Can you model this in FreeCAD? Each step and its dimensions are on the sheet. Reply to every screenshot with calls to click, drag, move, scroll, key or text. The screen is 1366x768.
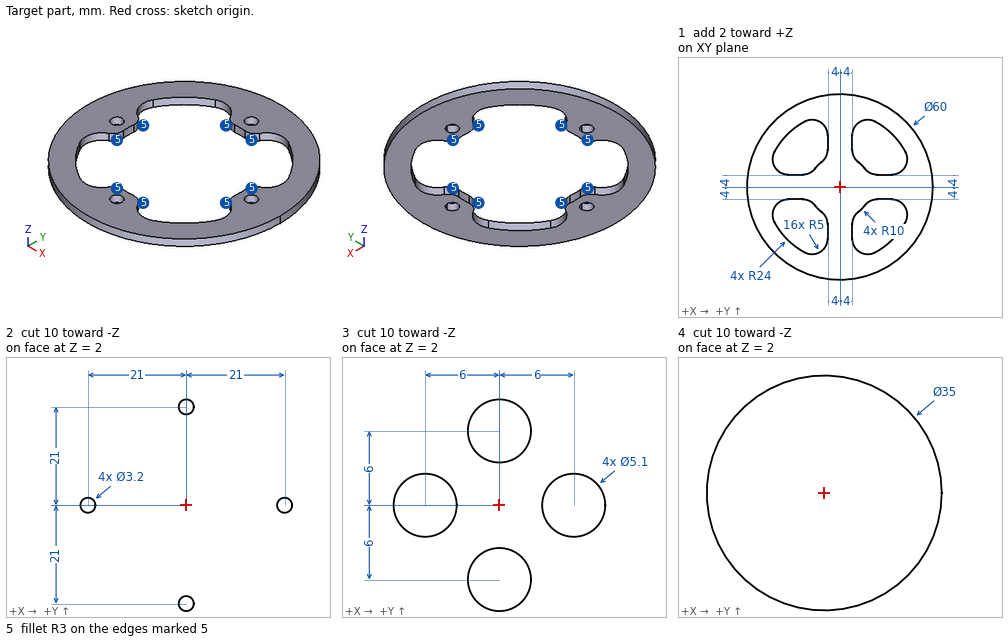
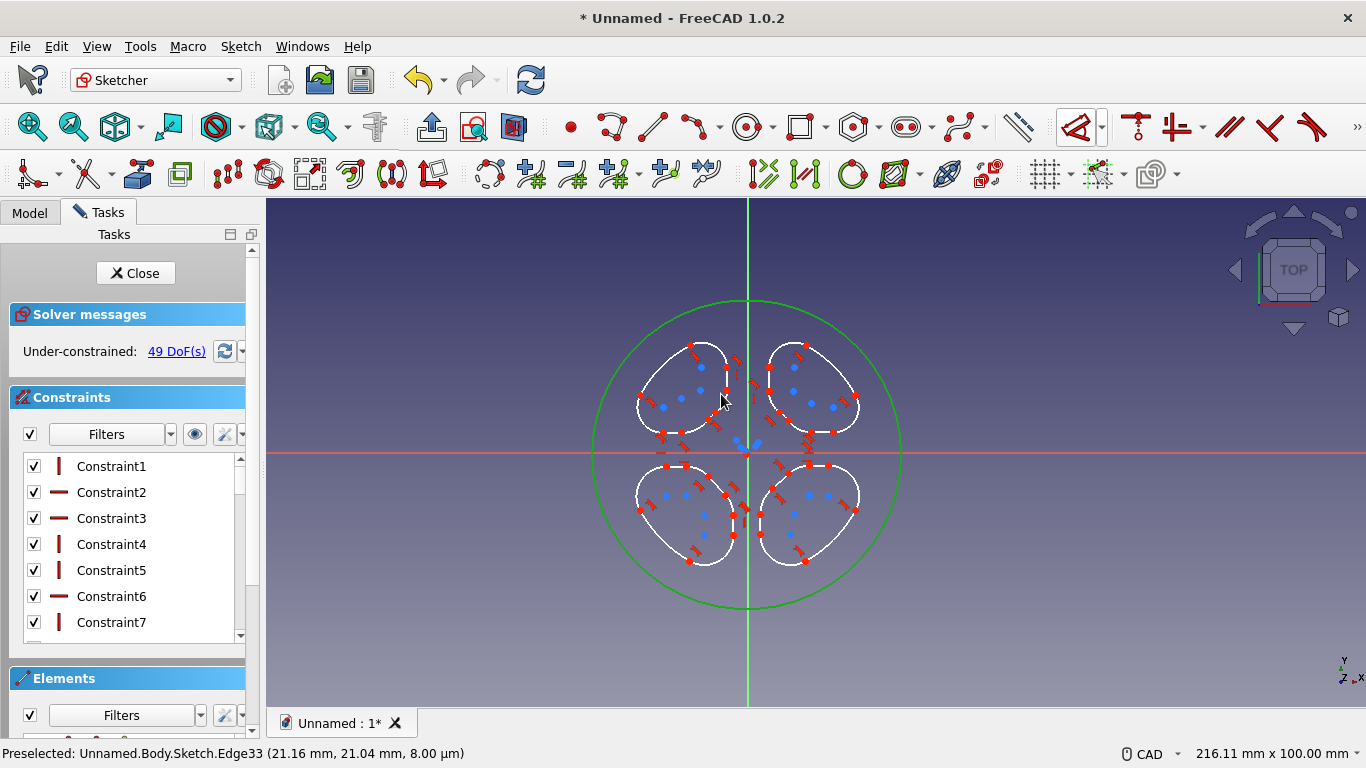
click(652, 529)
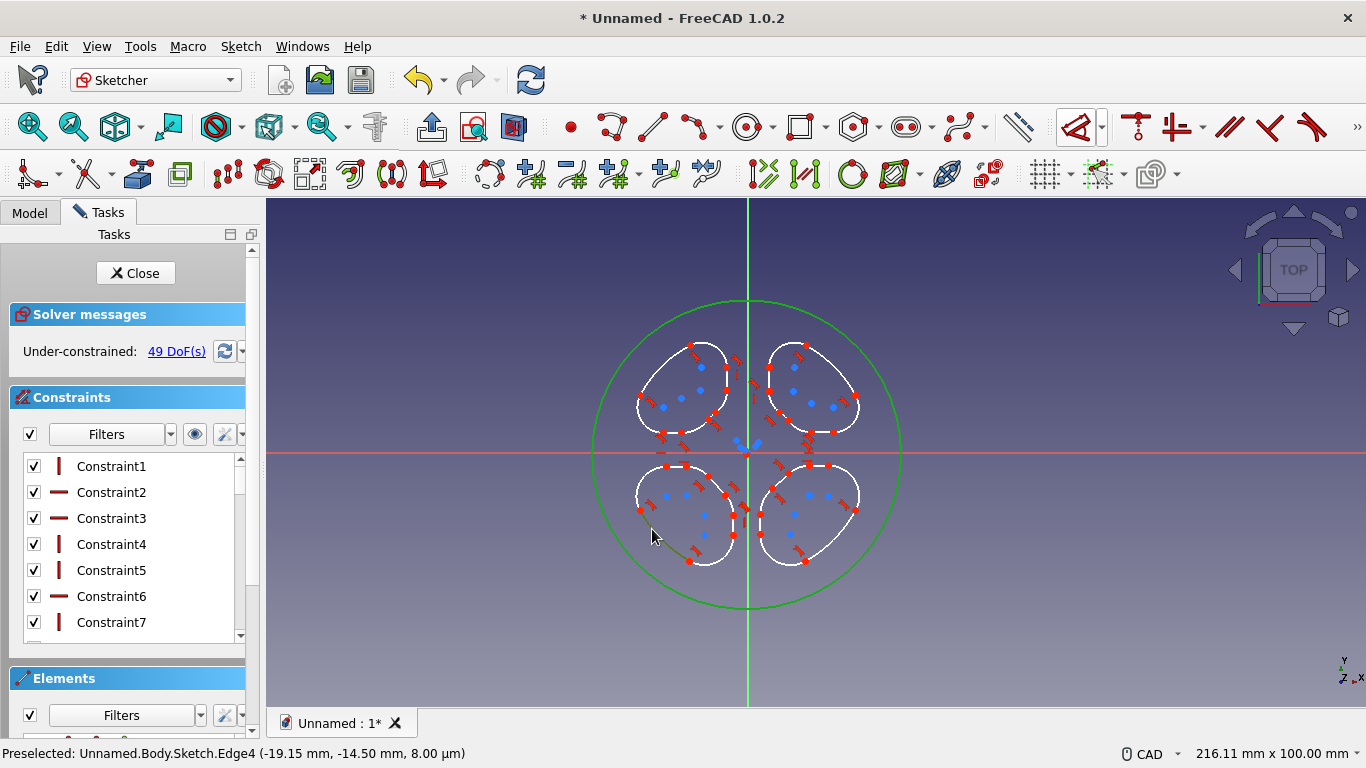
key(c)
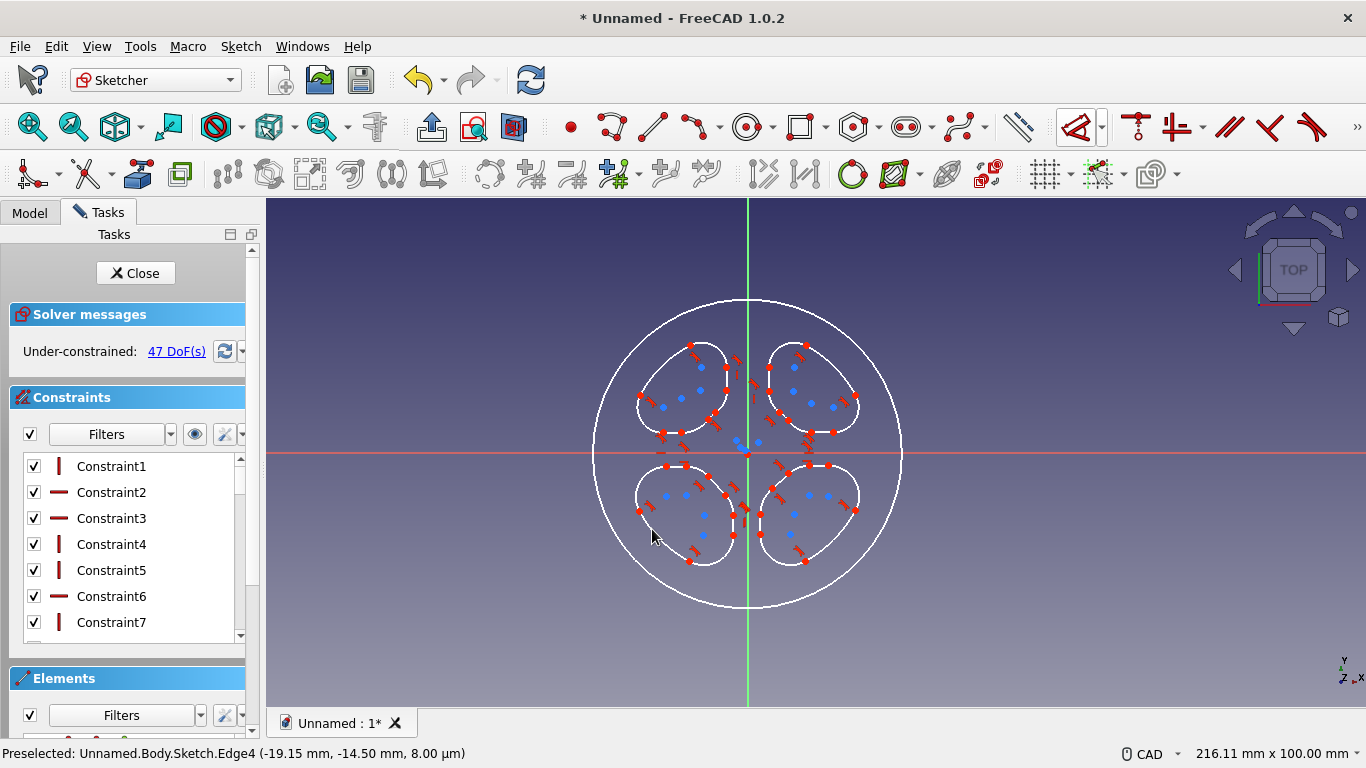
click(856, 344)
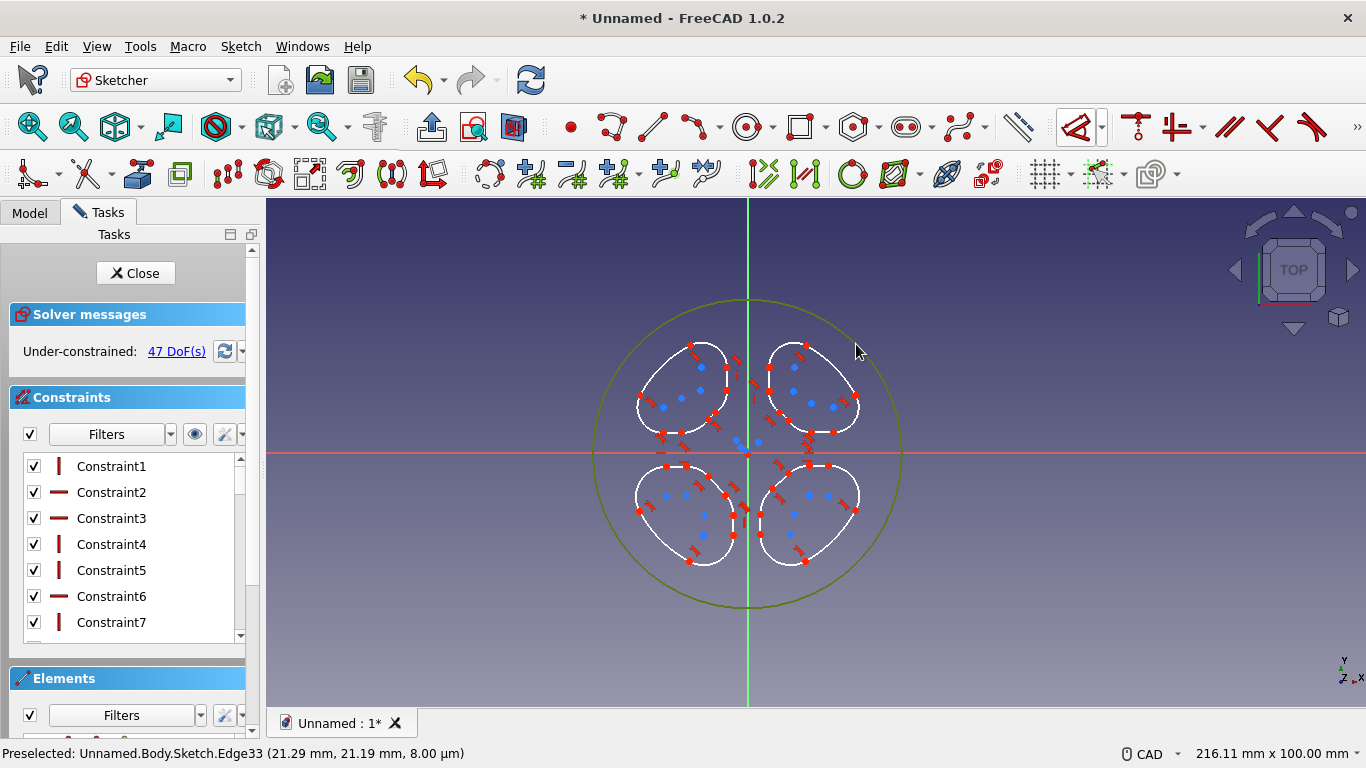
click(717, 486)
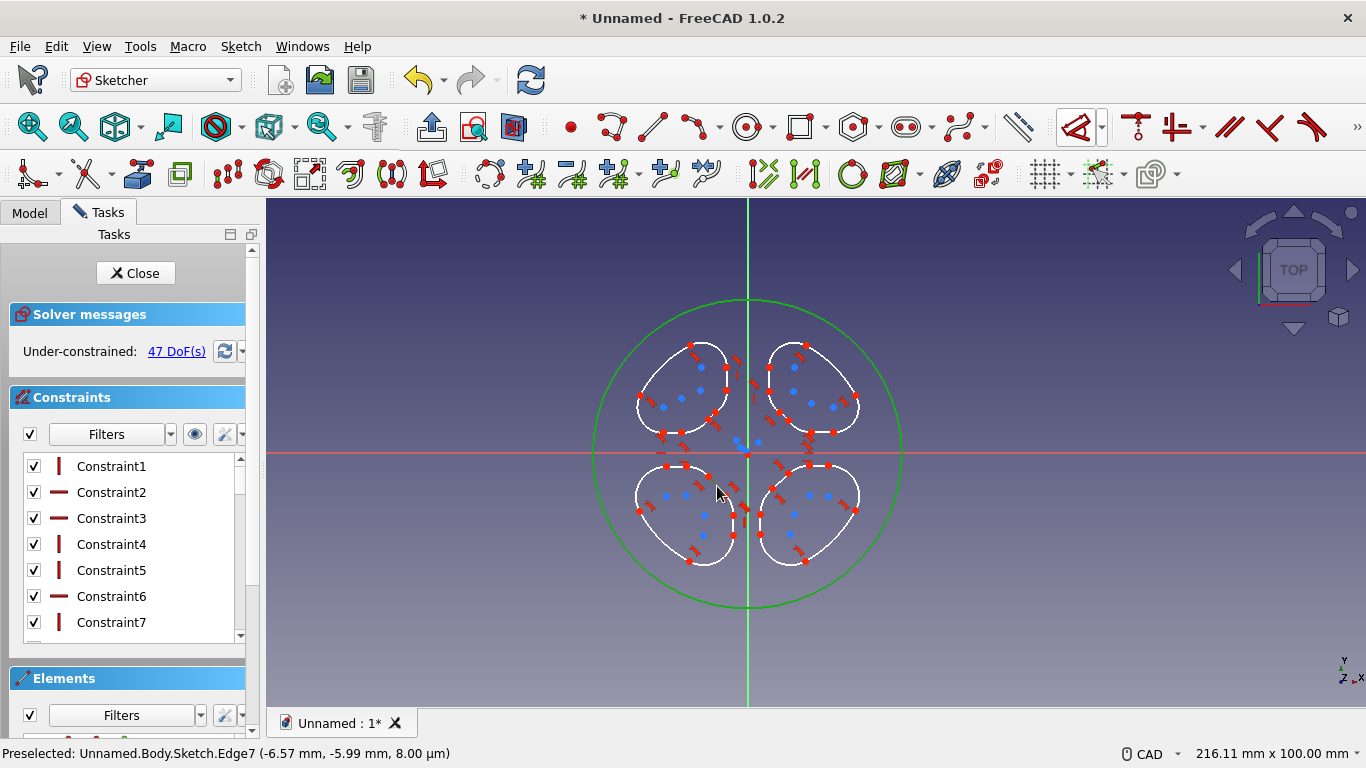
key(c)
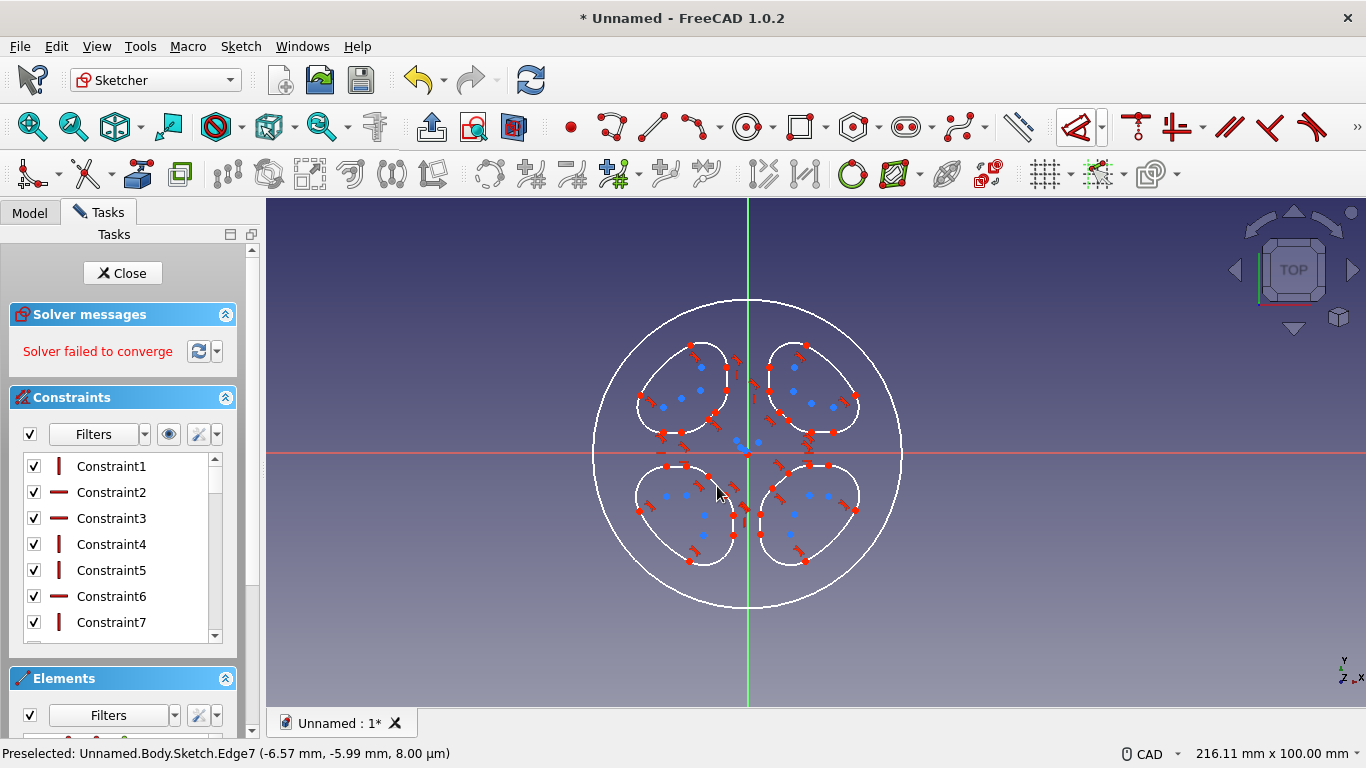
click(856, 344)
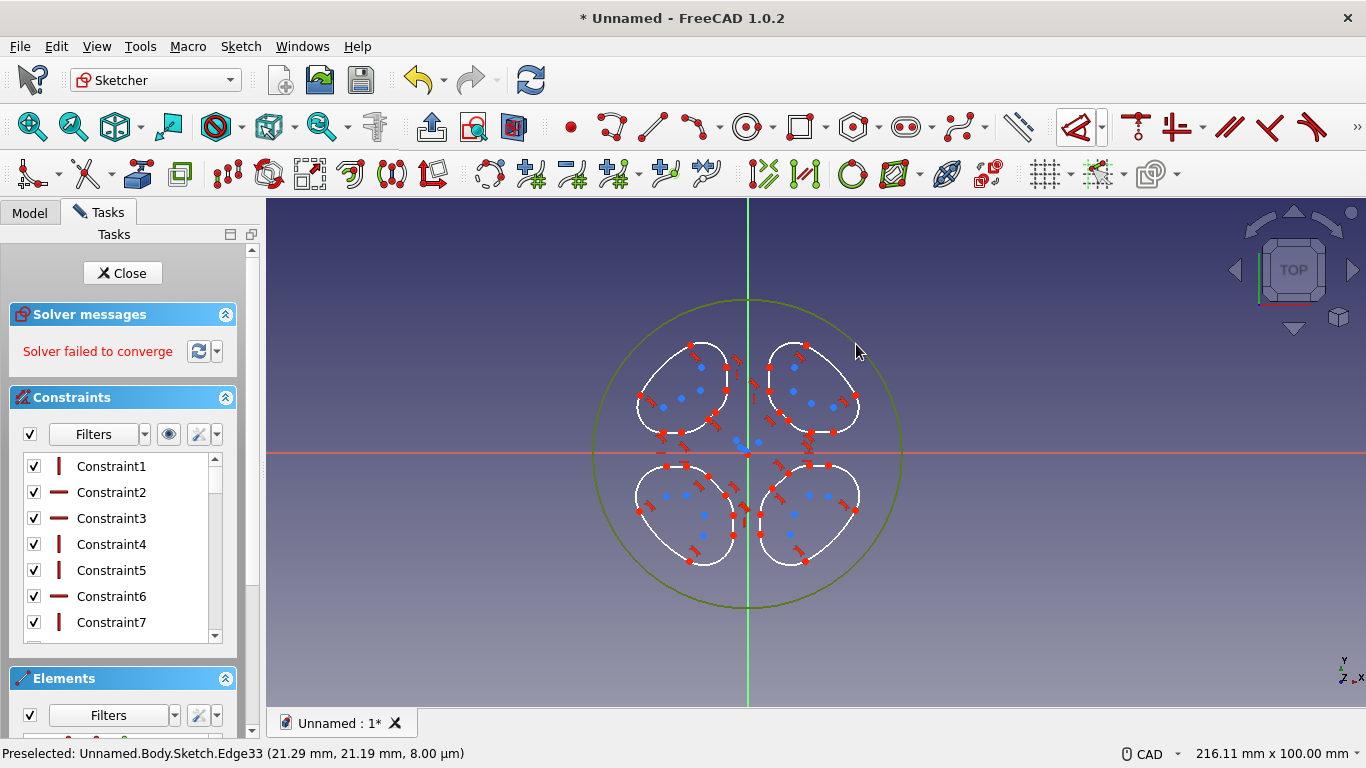
click(823, 549)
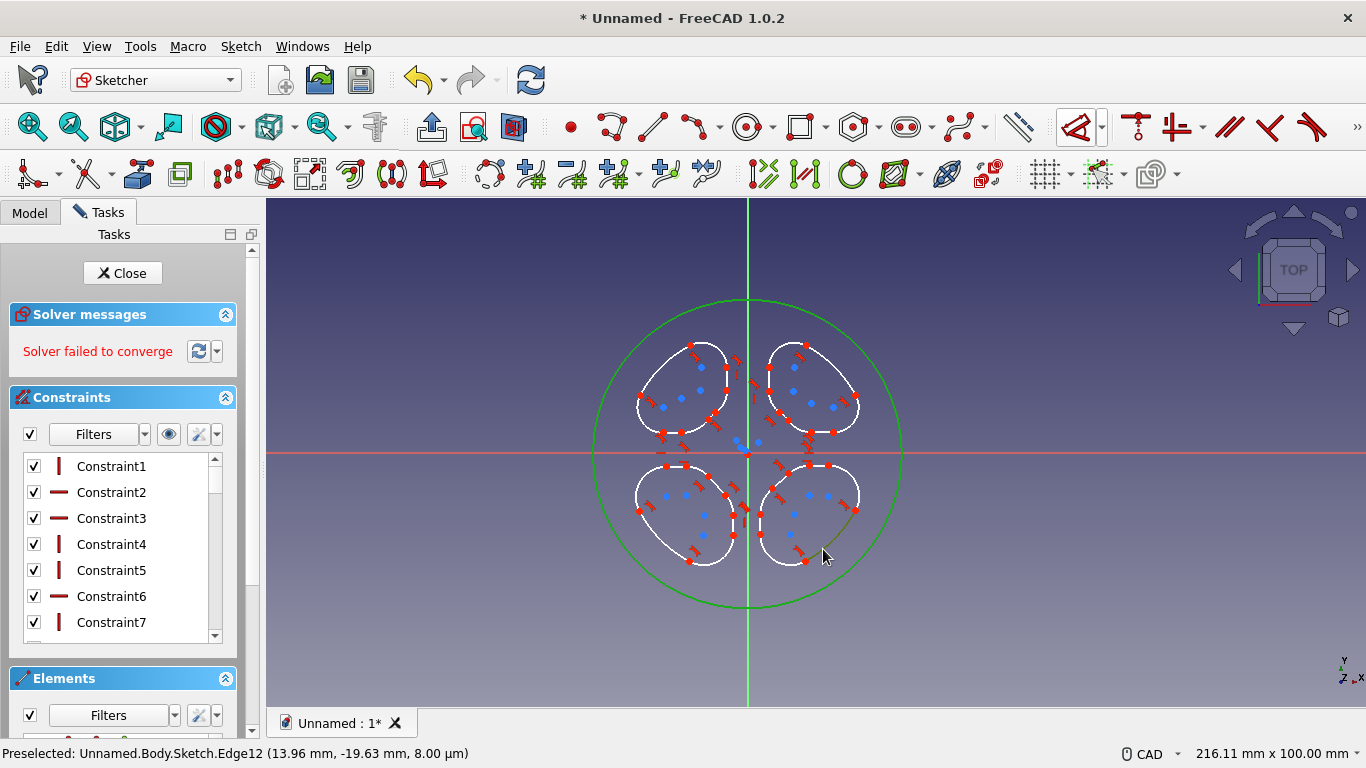
key(c)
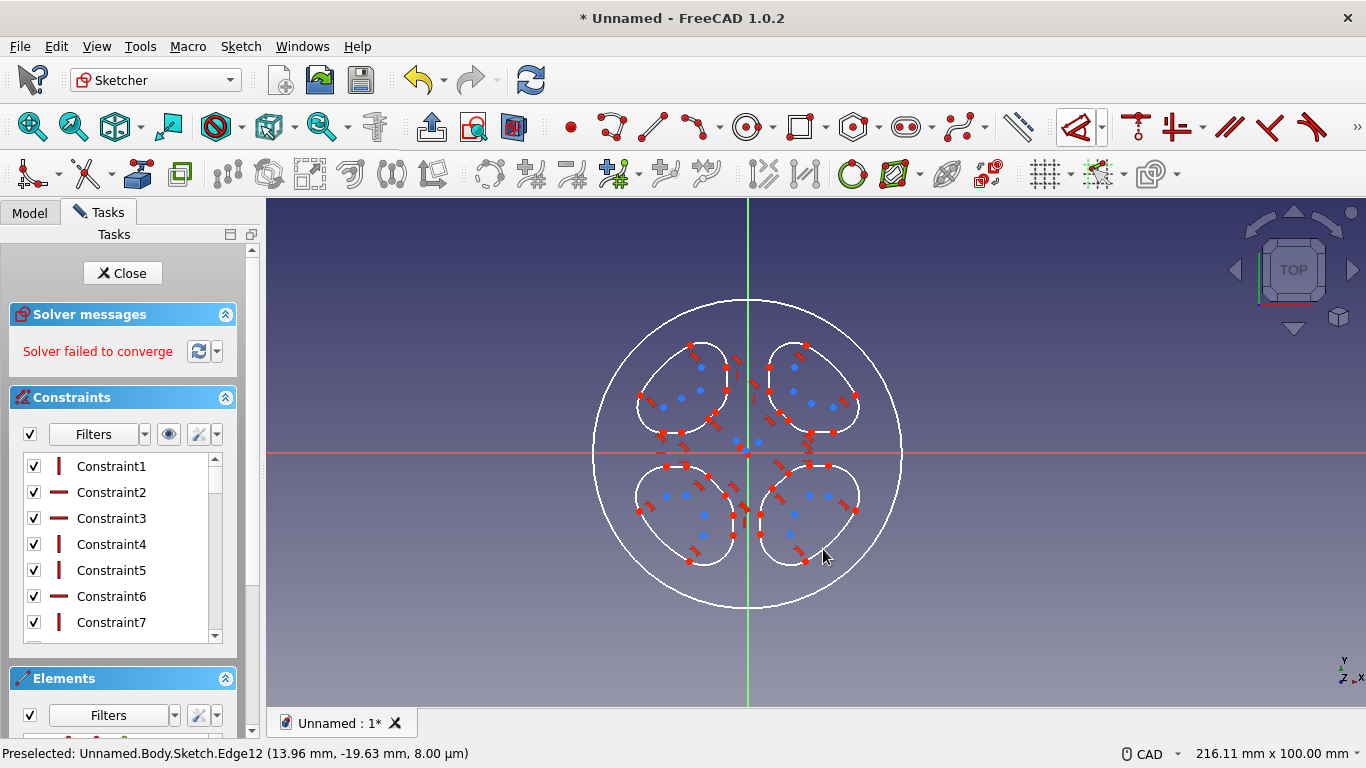
click(856, 344)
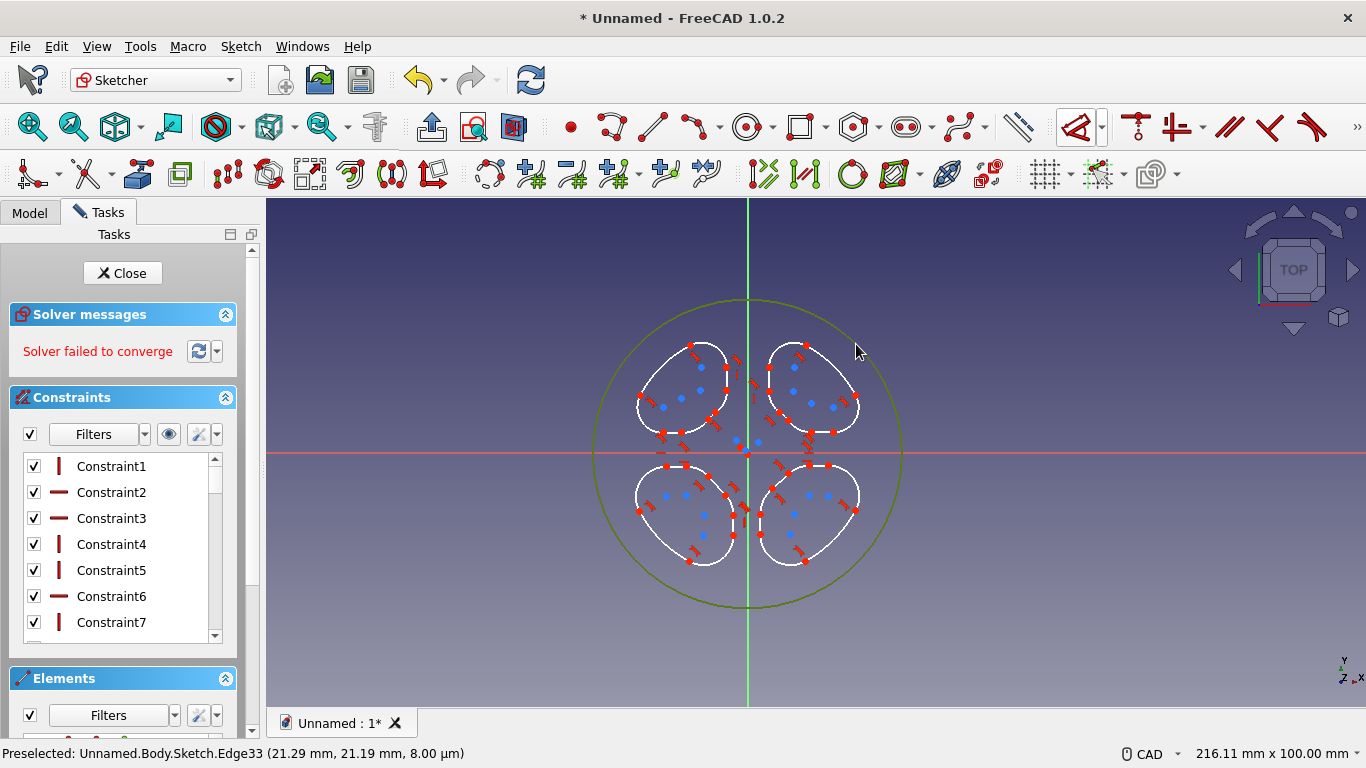
scroll(781, 482, up, 2)